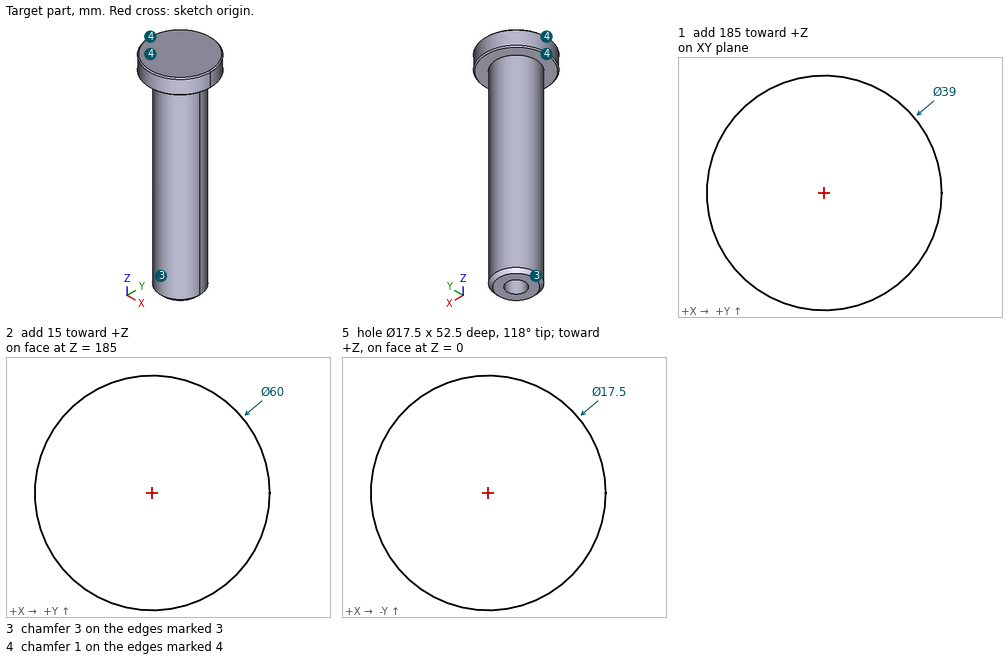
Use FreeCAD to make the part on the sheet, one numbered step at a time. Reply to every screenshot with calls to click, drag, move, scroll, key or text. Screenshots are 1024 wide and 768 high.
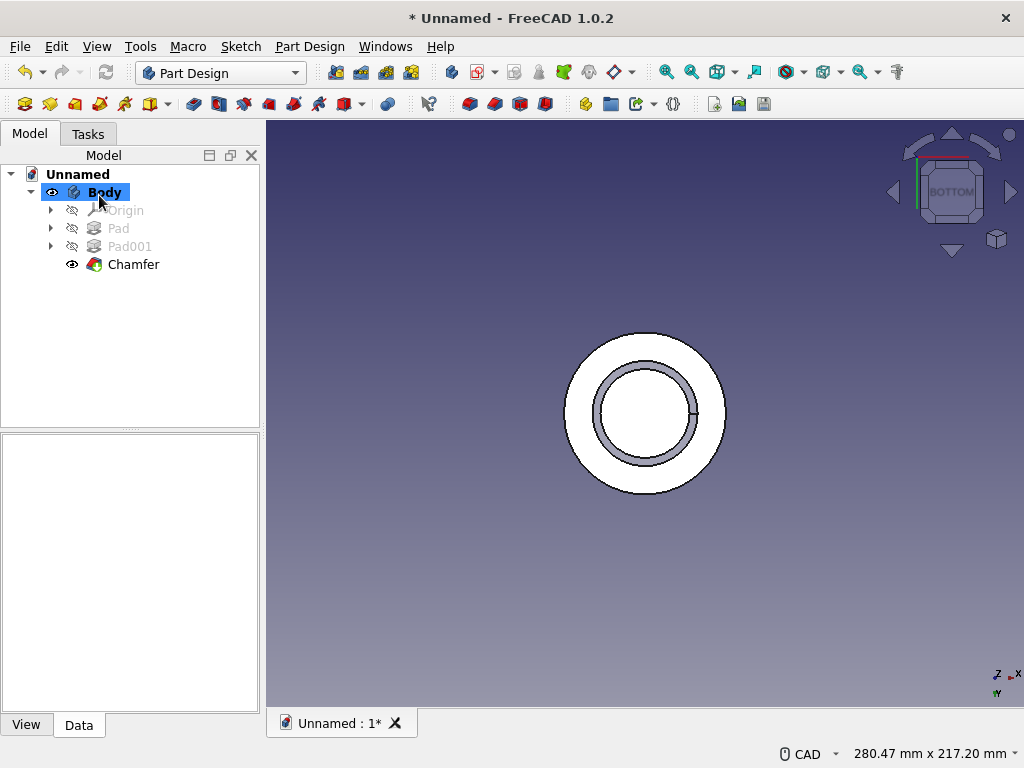
click(667, 72)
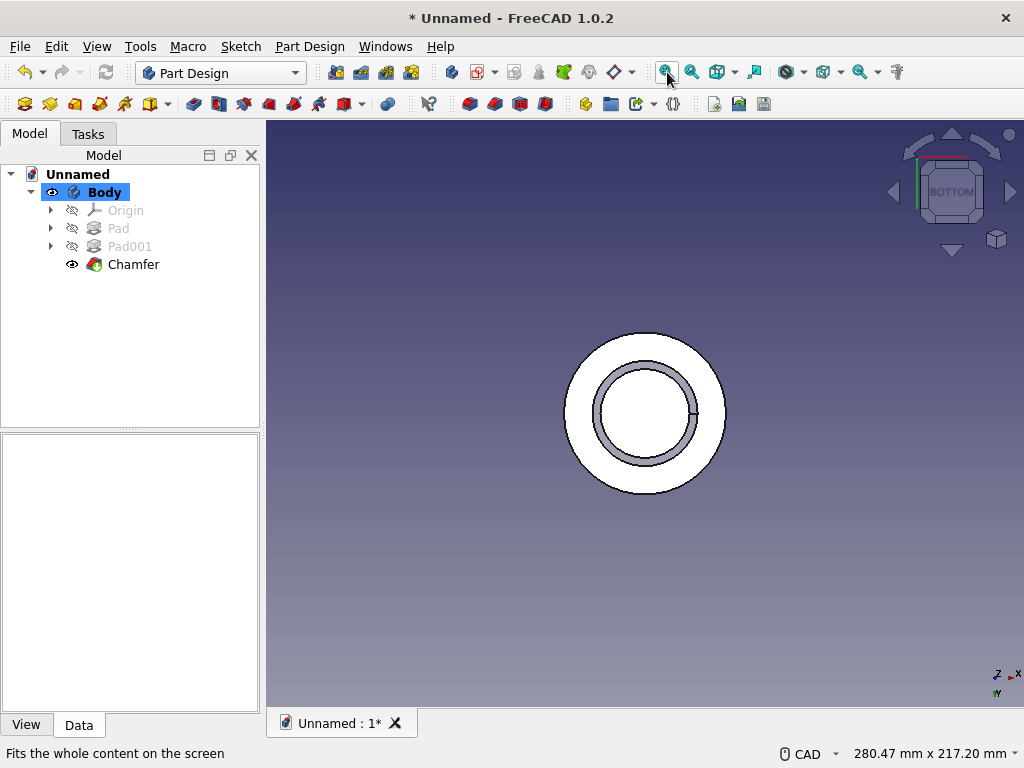
click(564, 412)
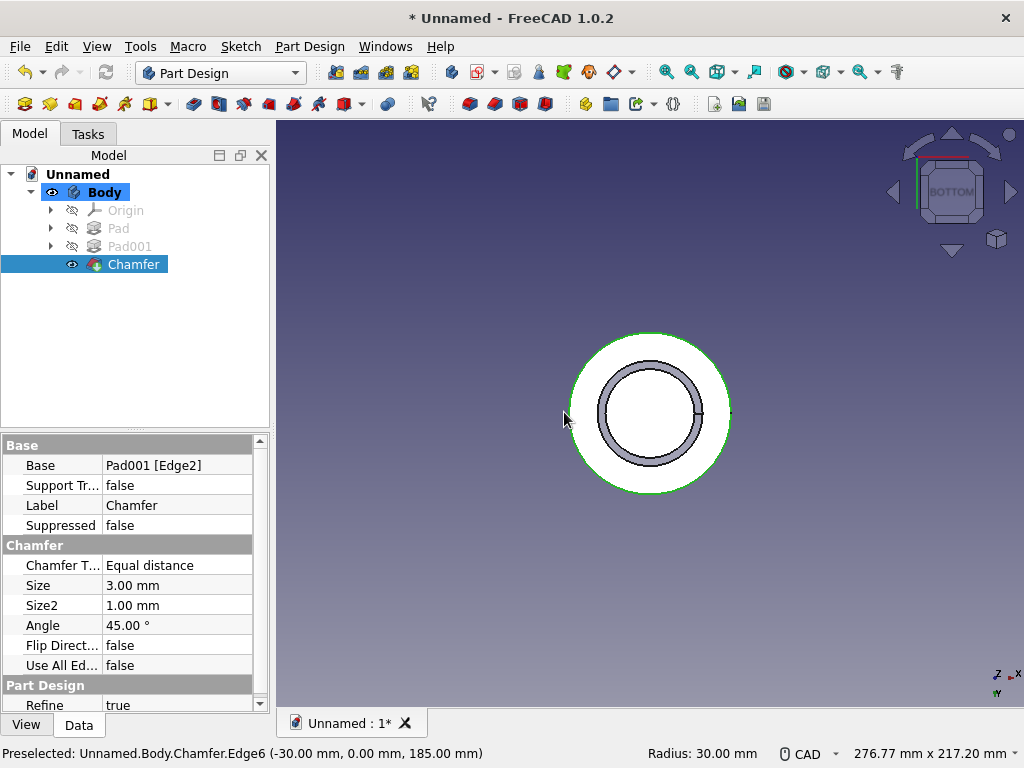
key(0)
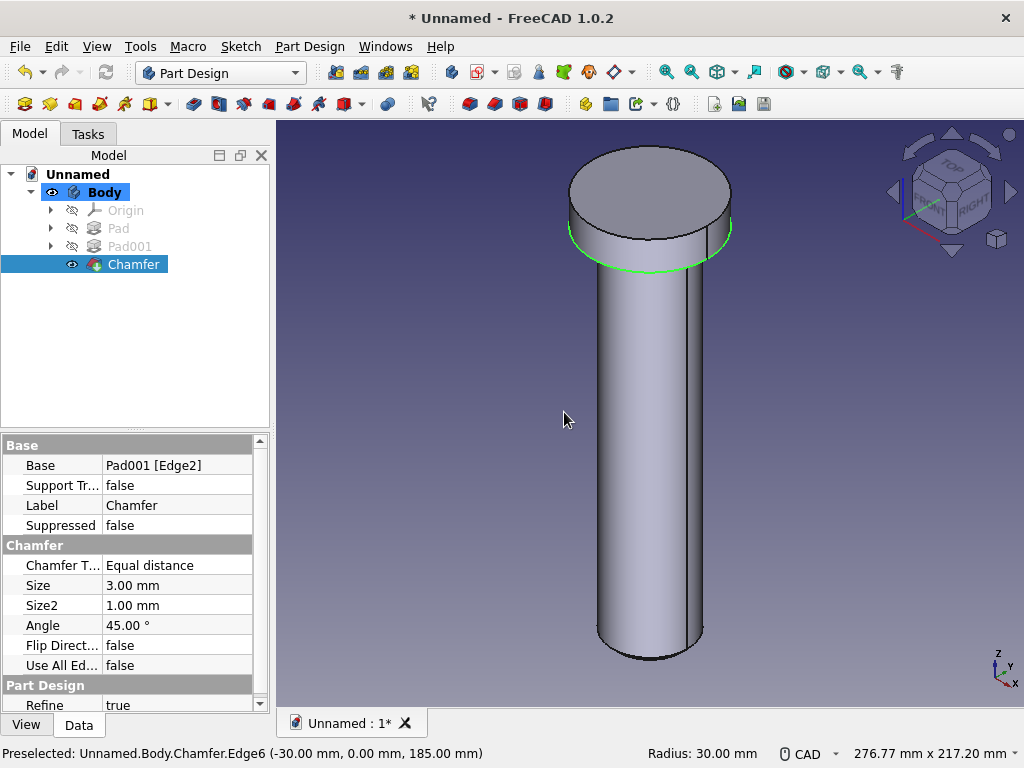
click(570, 185, ctrl)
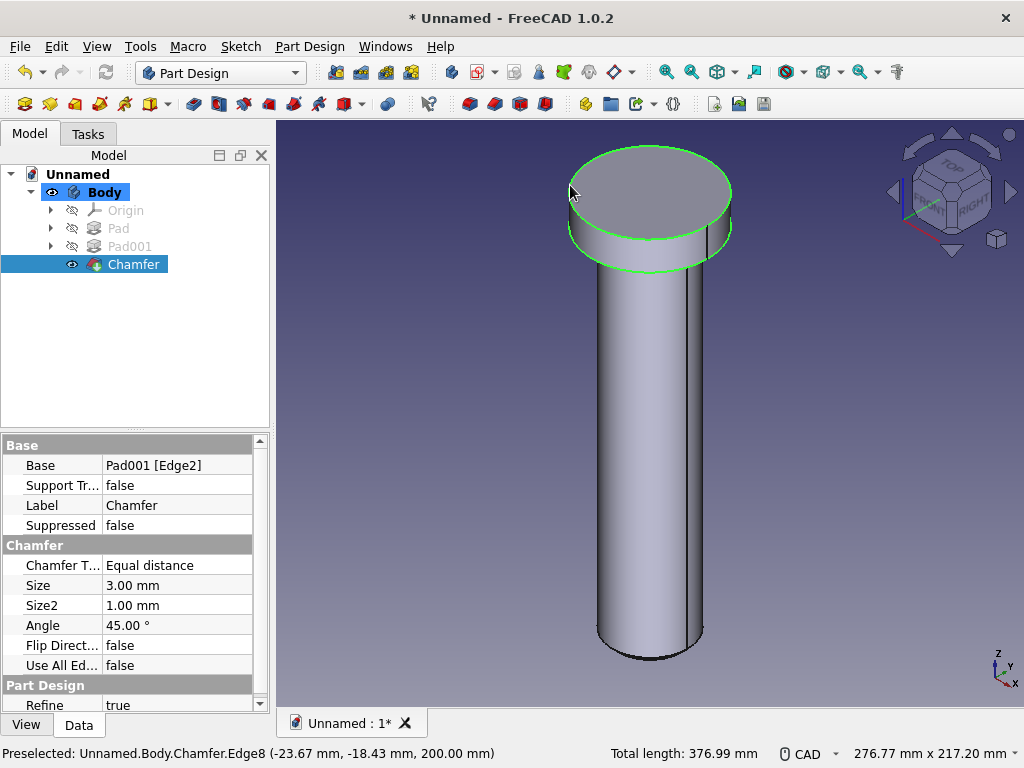
click(495, 104)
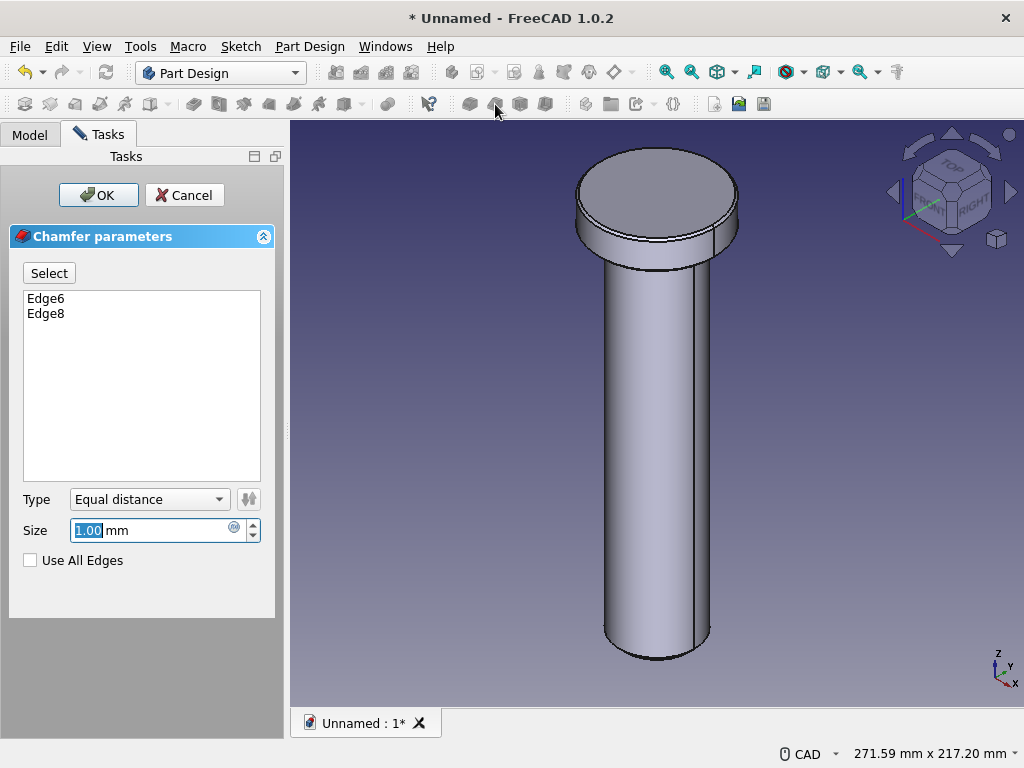
text(1)
key(Tab)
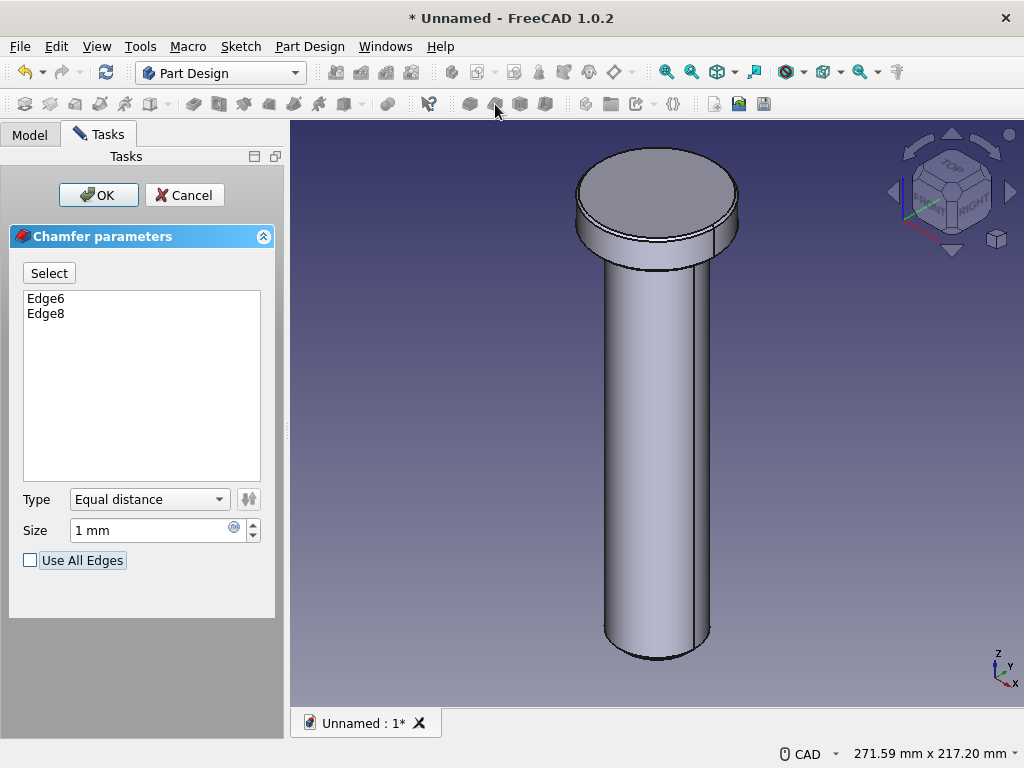
click(99, 195)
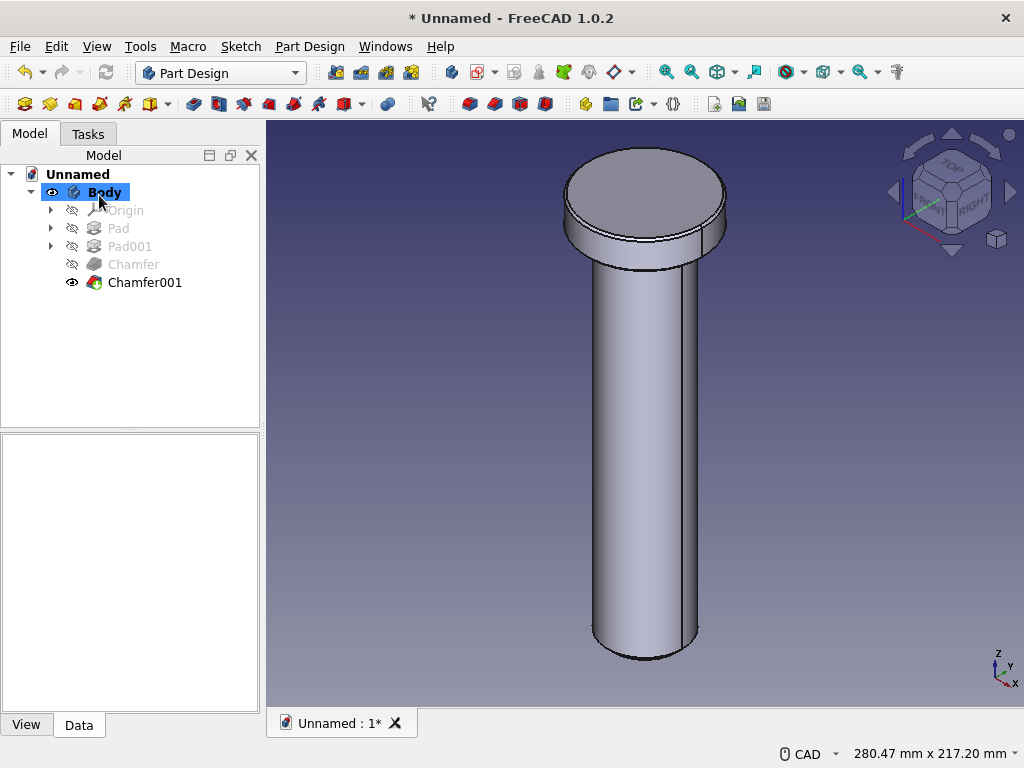
key(5)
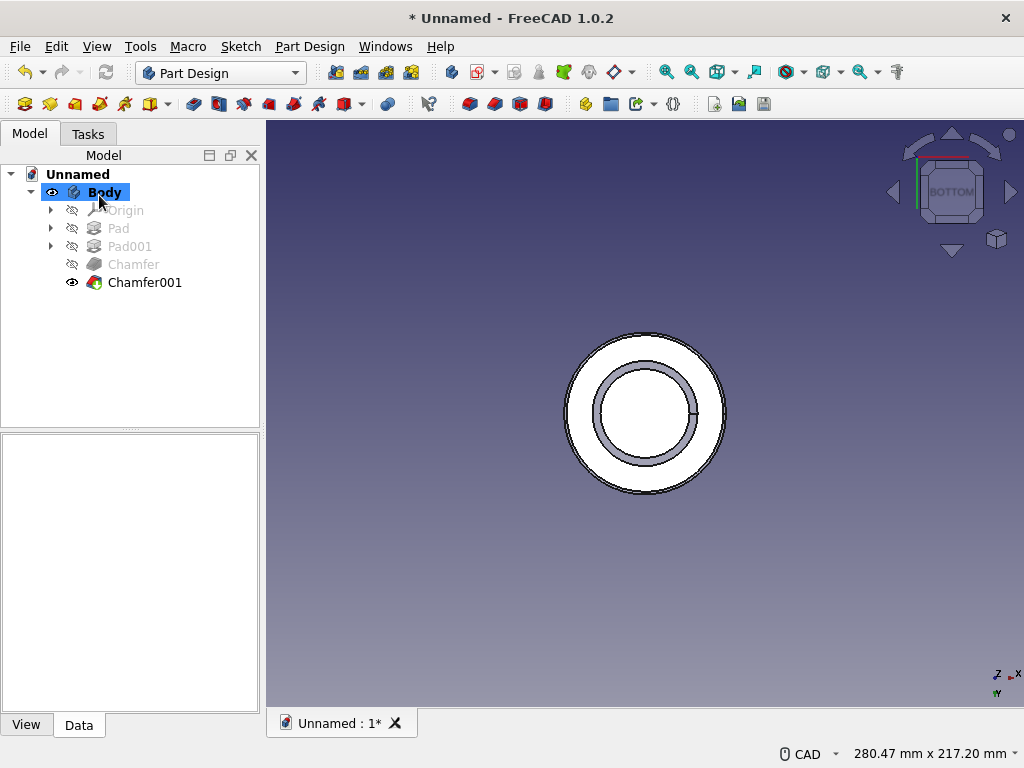
click(667, 72)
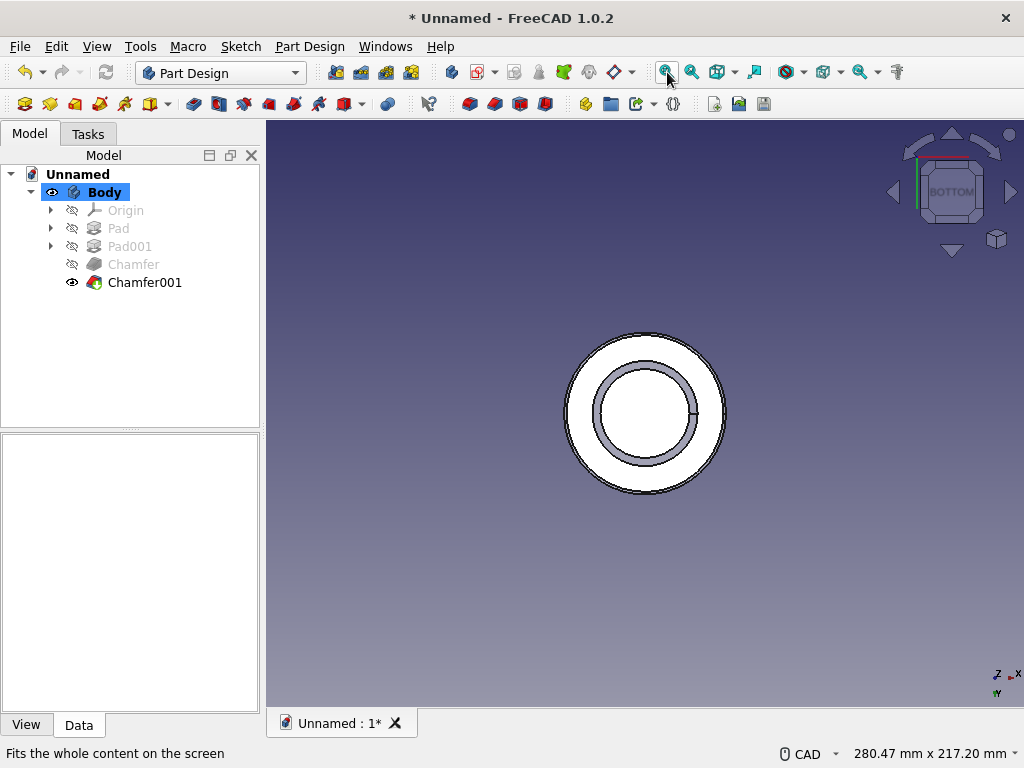
click(645, 412)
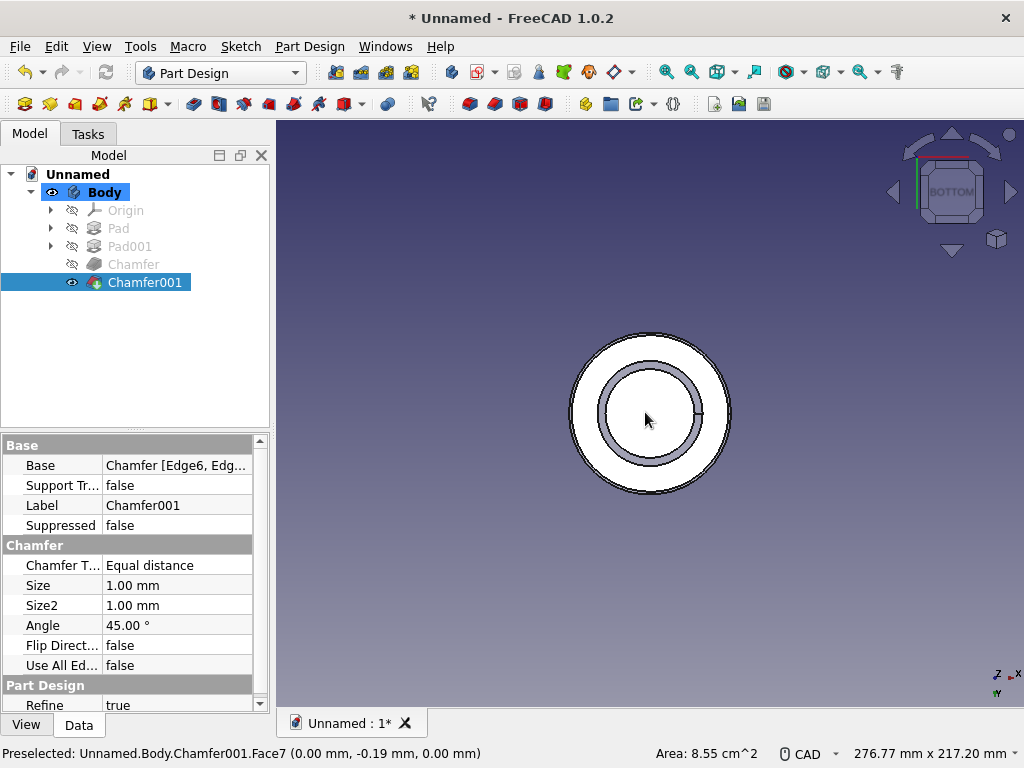
click(476, 72)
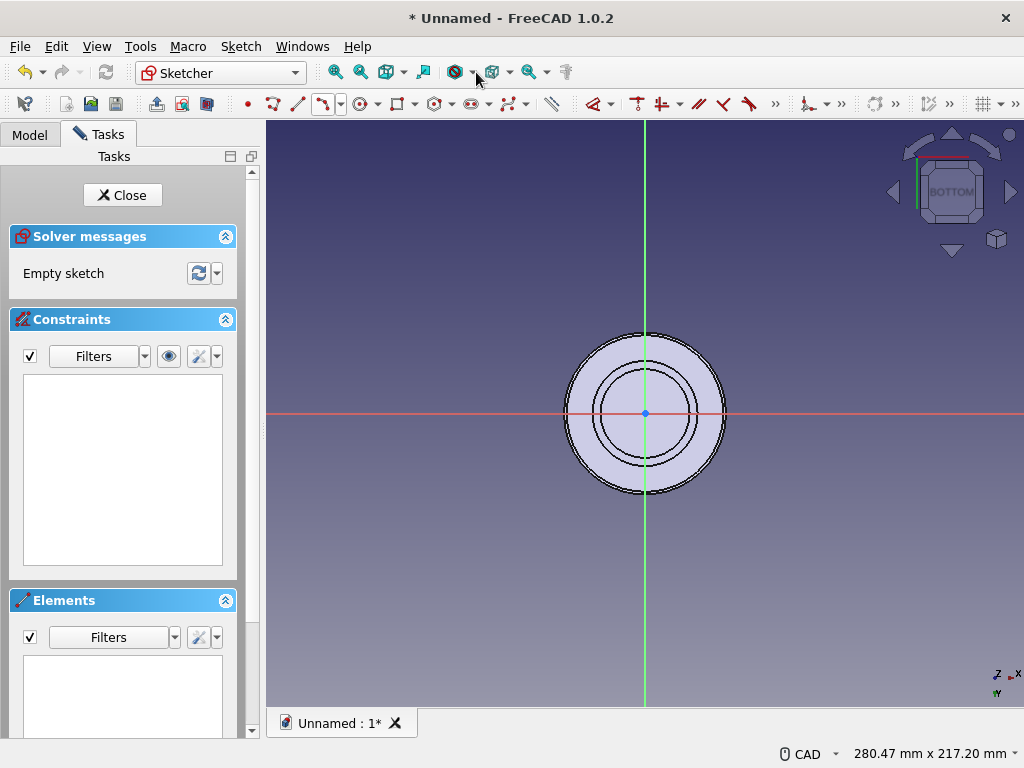
scroll(656, 414, up, 10)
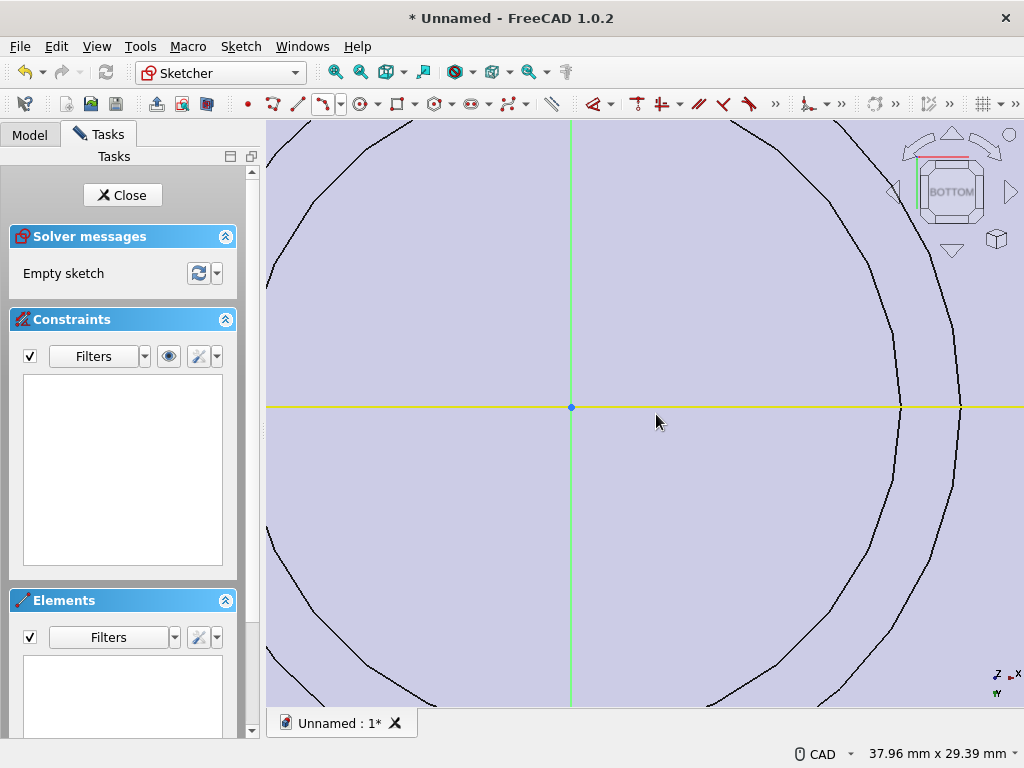
click(360, 104)